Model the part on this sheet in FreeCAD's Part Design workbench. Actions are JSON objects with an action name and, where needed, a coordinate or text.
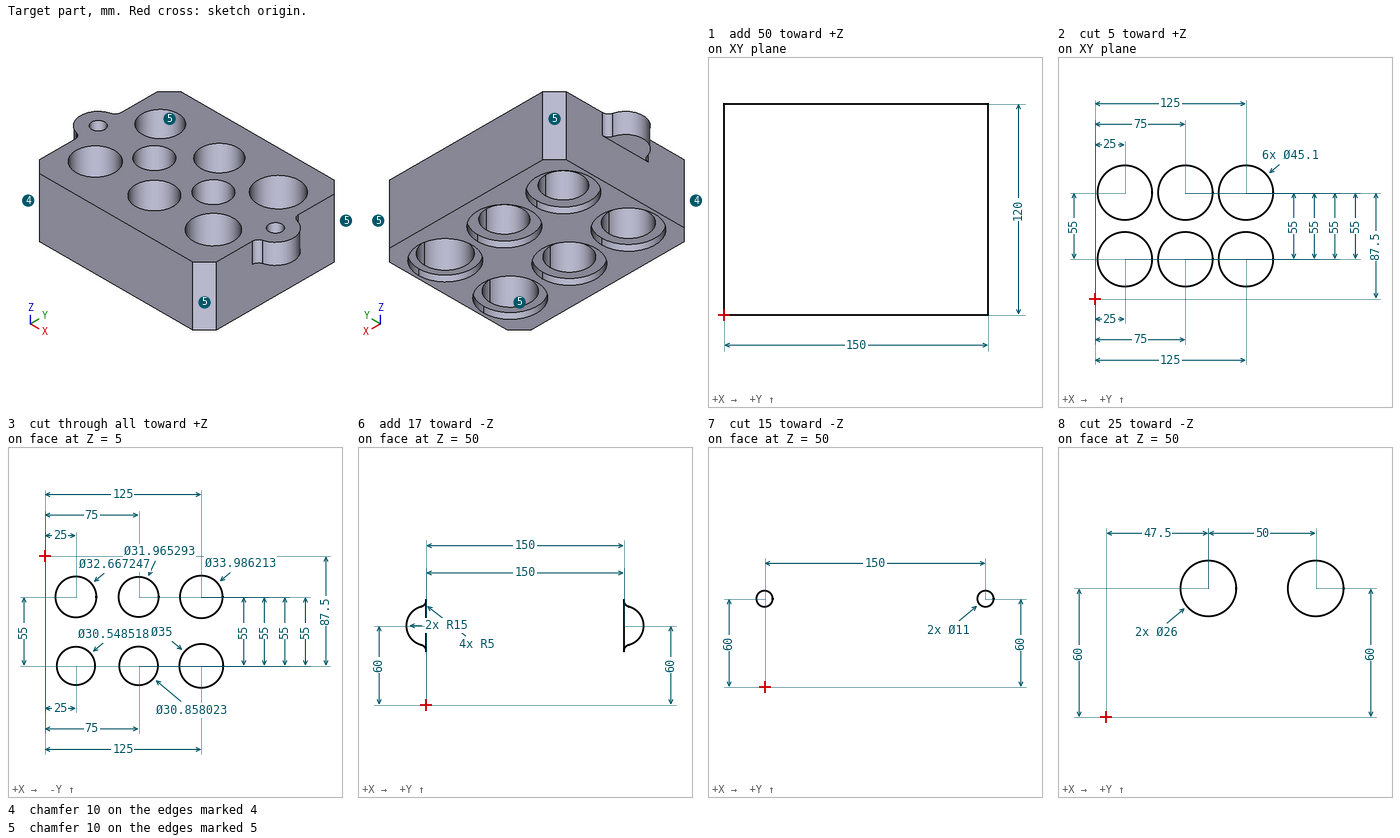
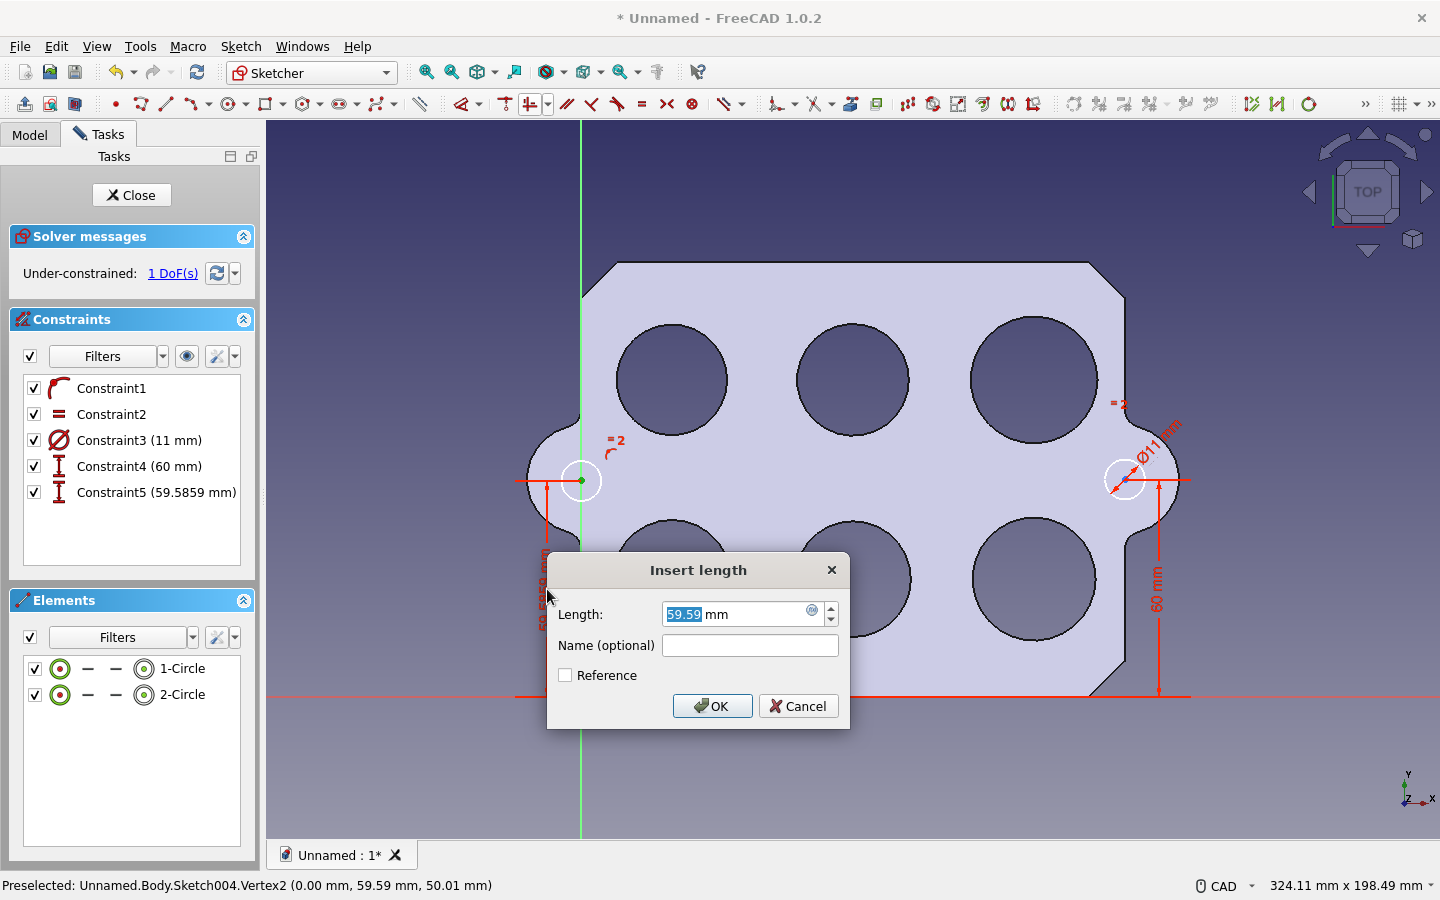
{"action": "type", "text": "60"}
{"action": "key", "text": "Return"}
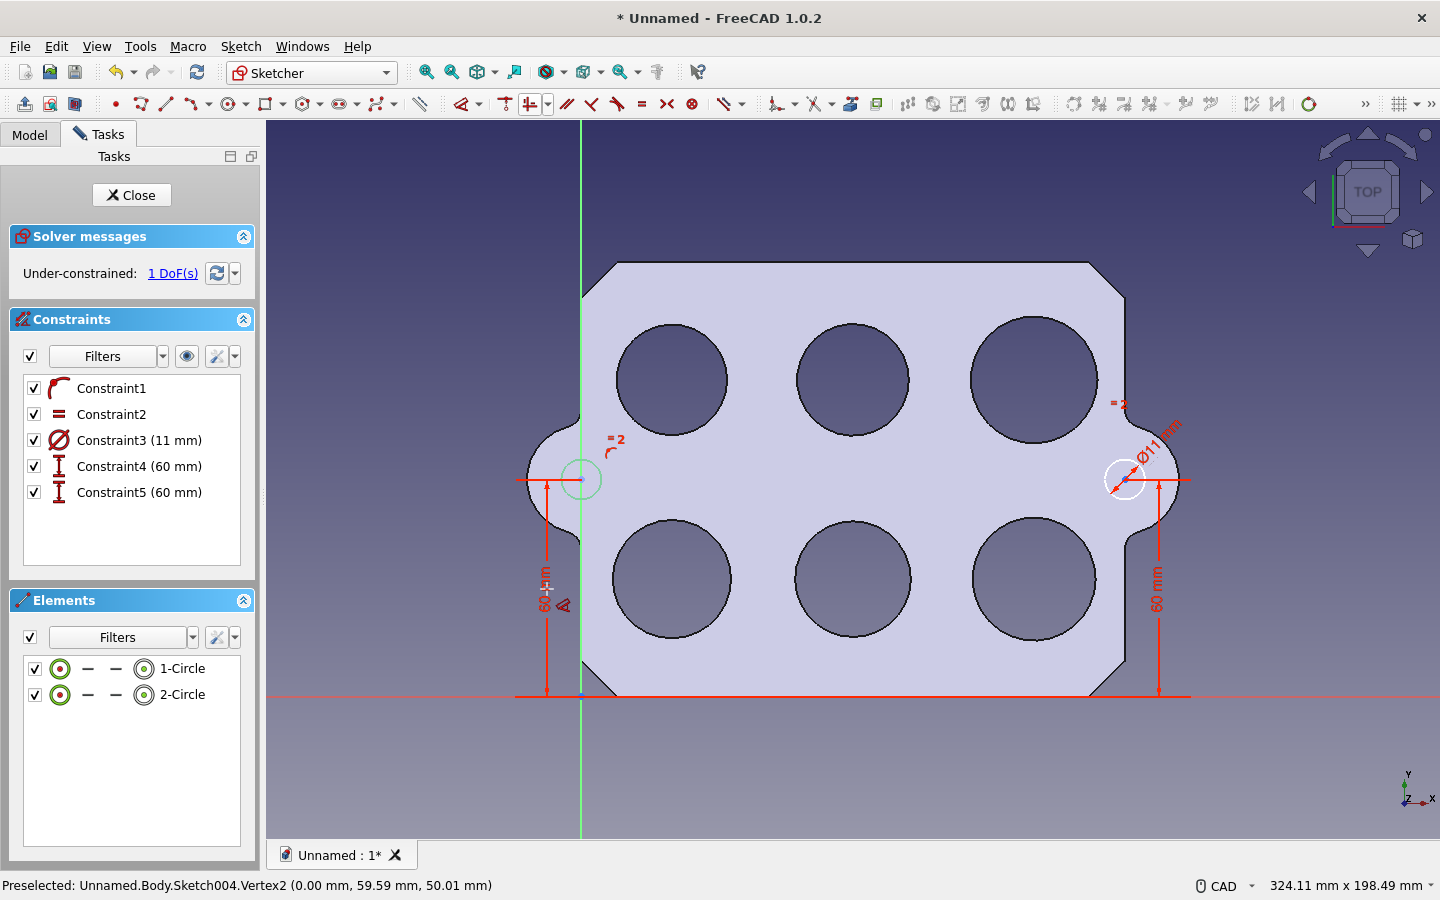
{"action": "left_click", "coordinate": [1125, 480]}
{"action": "left_click", "coordinate": [853, 731]}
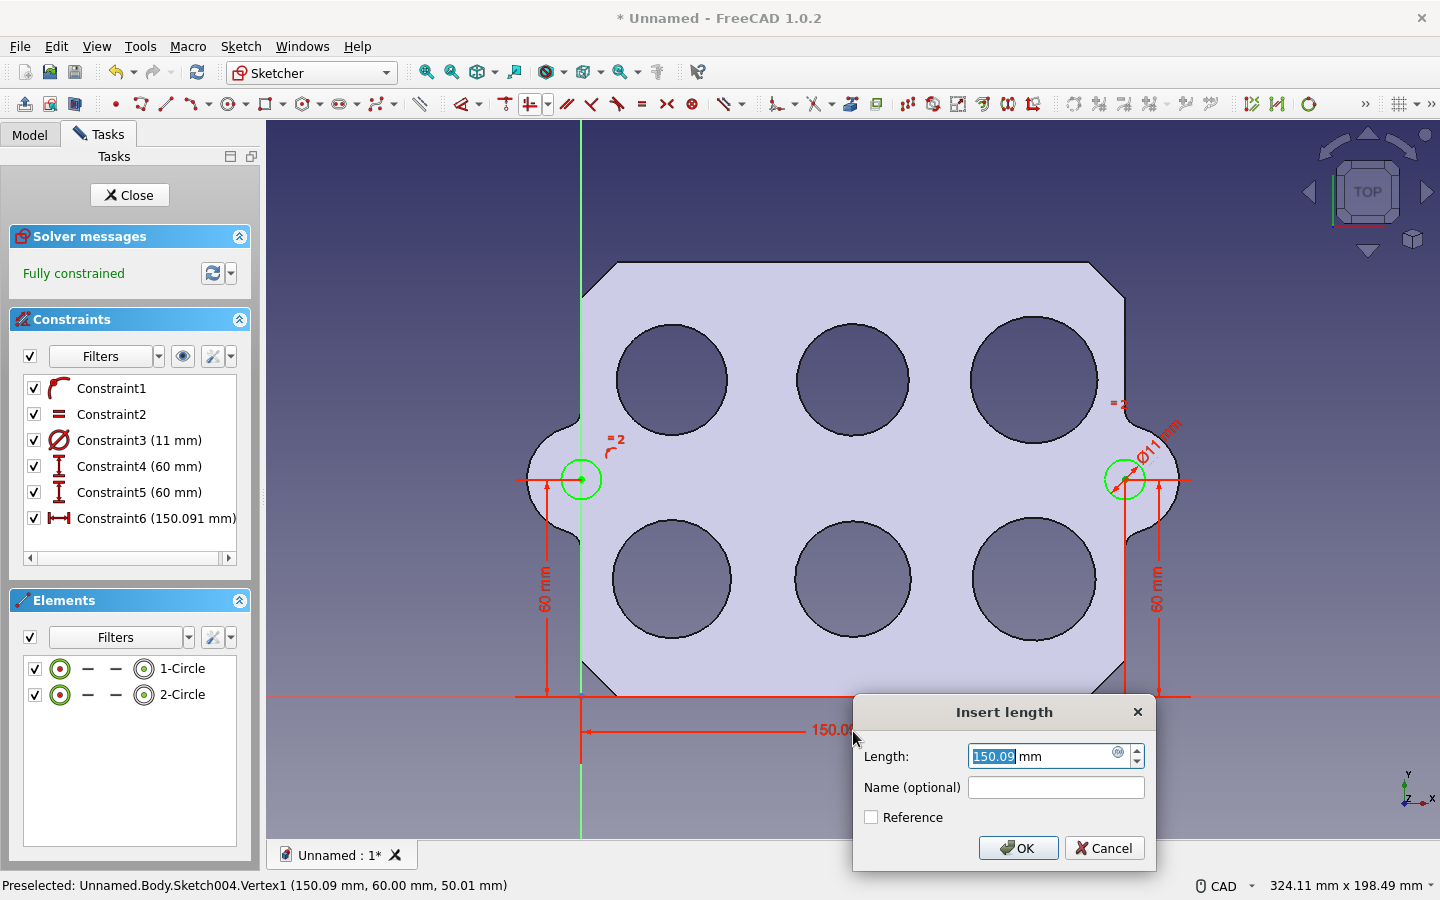
{"action": "type", "text": "150"}
{"action": "key", "text": "Return"}
{"action": "key", "text": "Escape"}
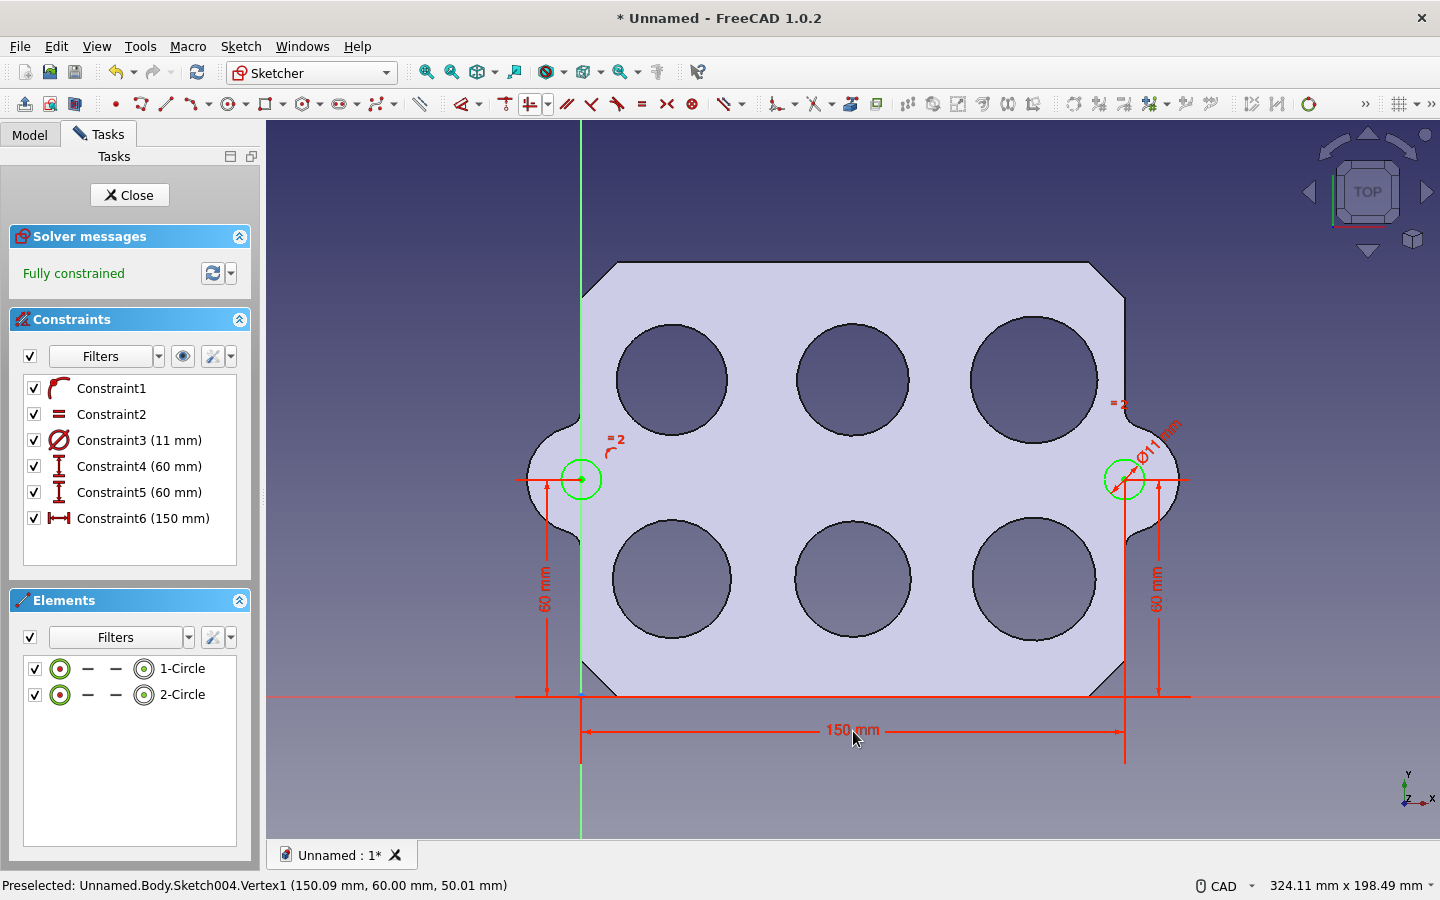
{"action": "left_click", "coordinate": [130, 195]}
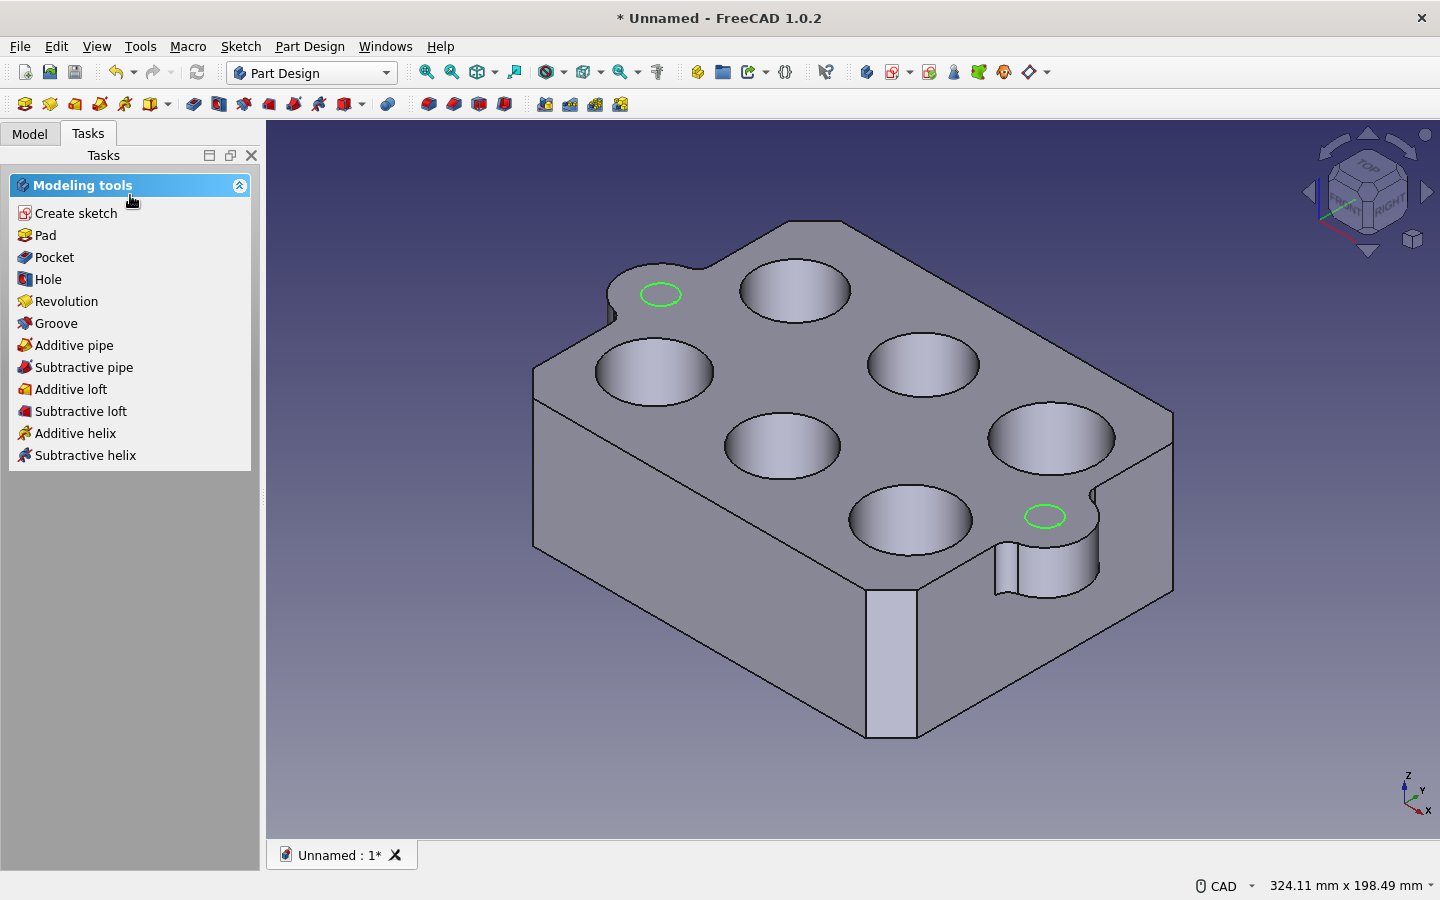
{"action": "left_click", "coordinate": [194, 104]}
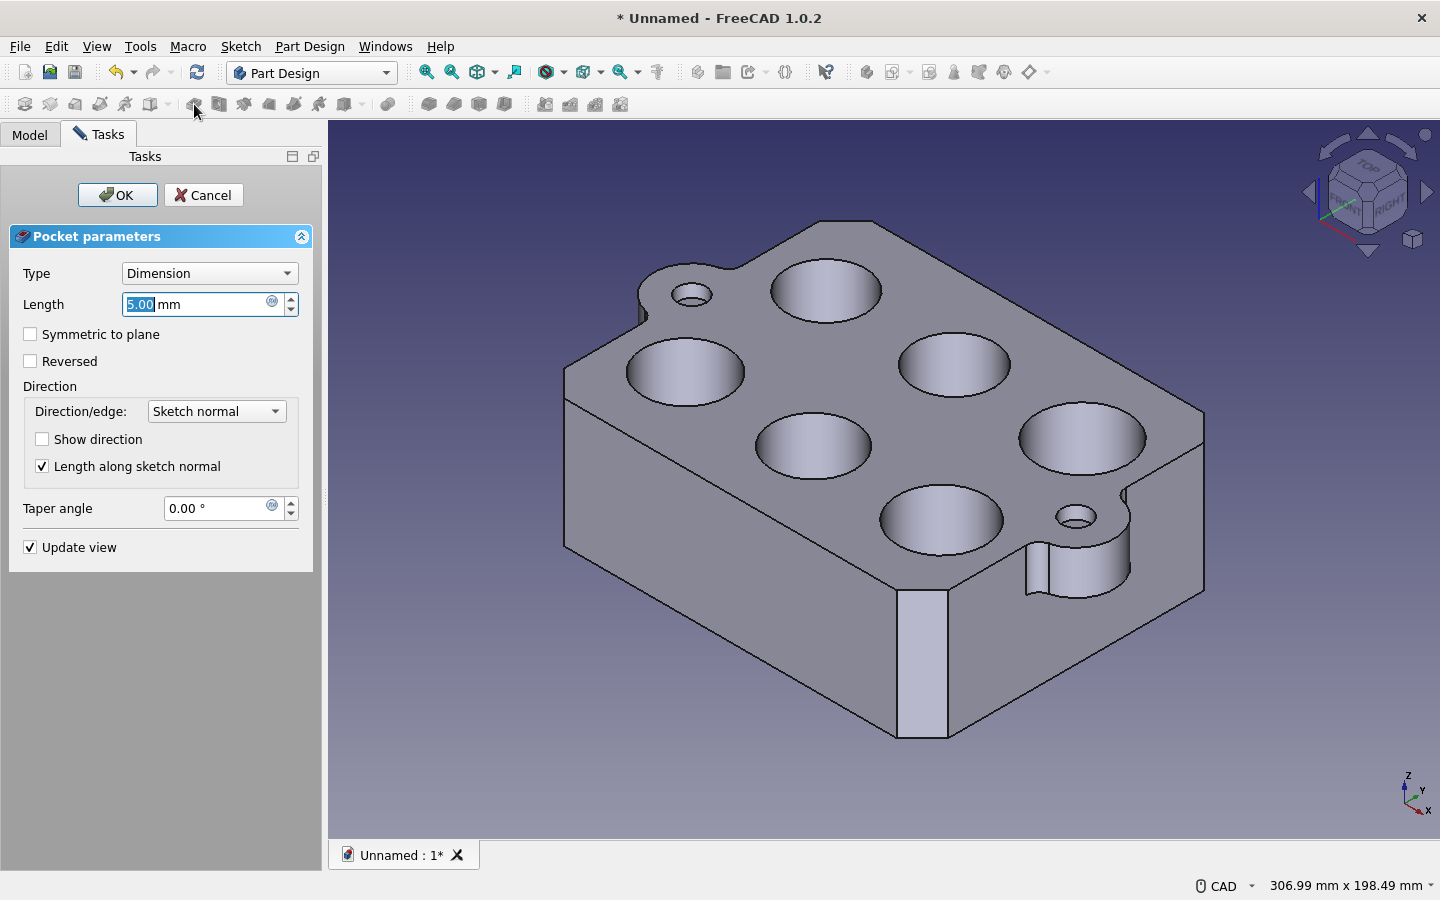
{"action": "type", "text": "15"}
{"action": "key", "text": "Tab"}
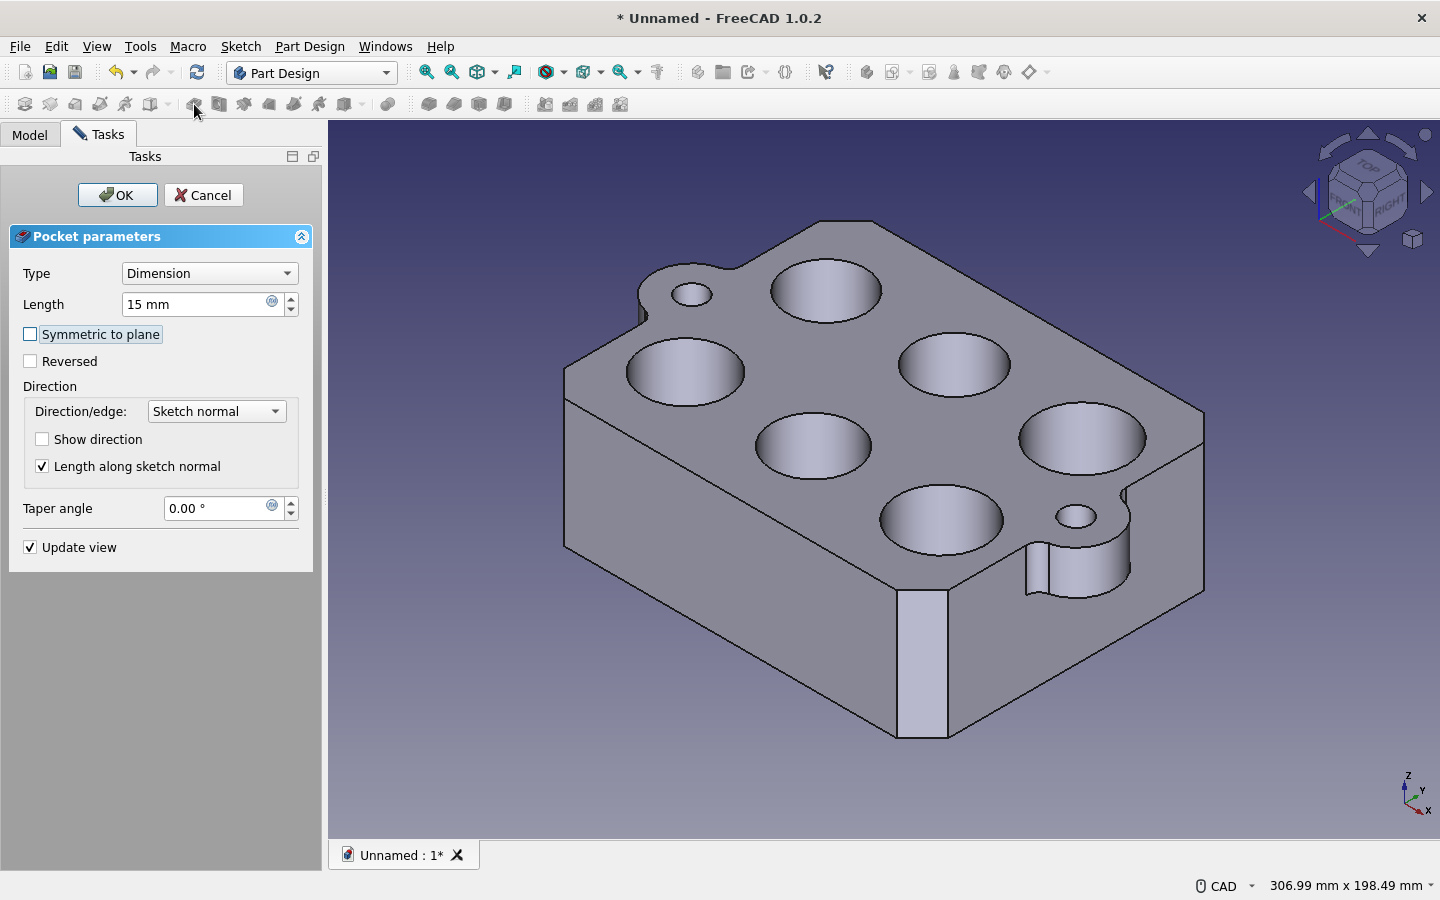
{"action": "left_click", "coordinate": [118, 195]}